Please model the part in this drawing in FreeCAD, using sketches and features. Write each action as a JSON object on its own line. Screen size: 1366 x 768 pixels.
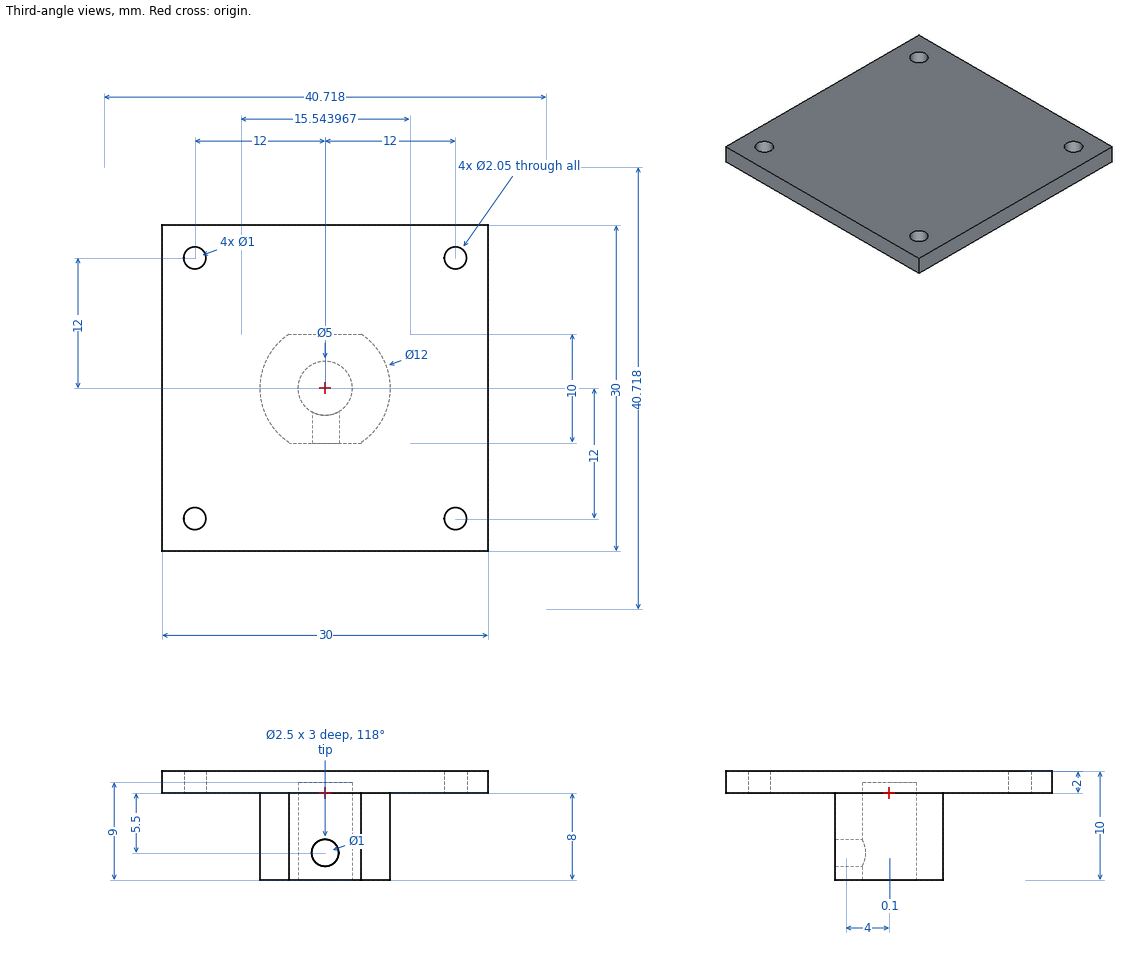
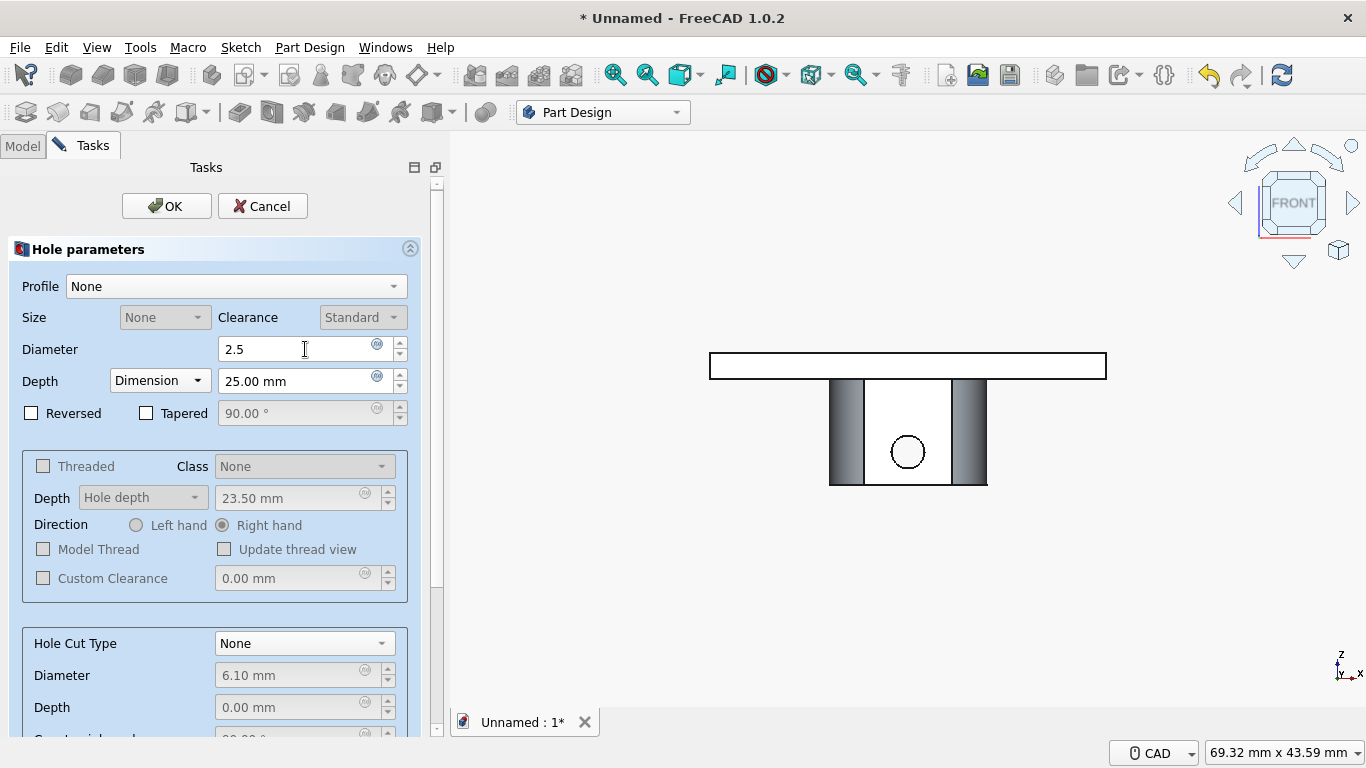
{"action": "triple_click", "coordinate": [305, 381]}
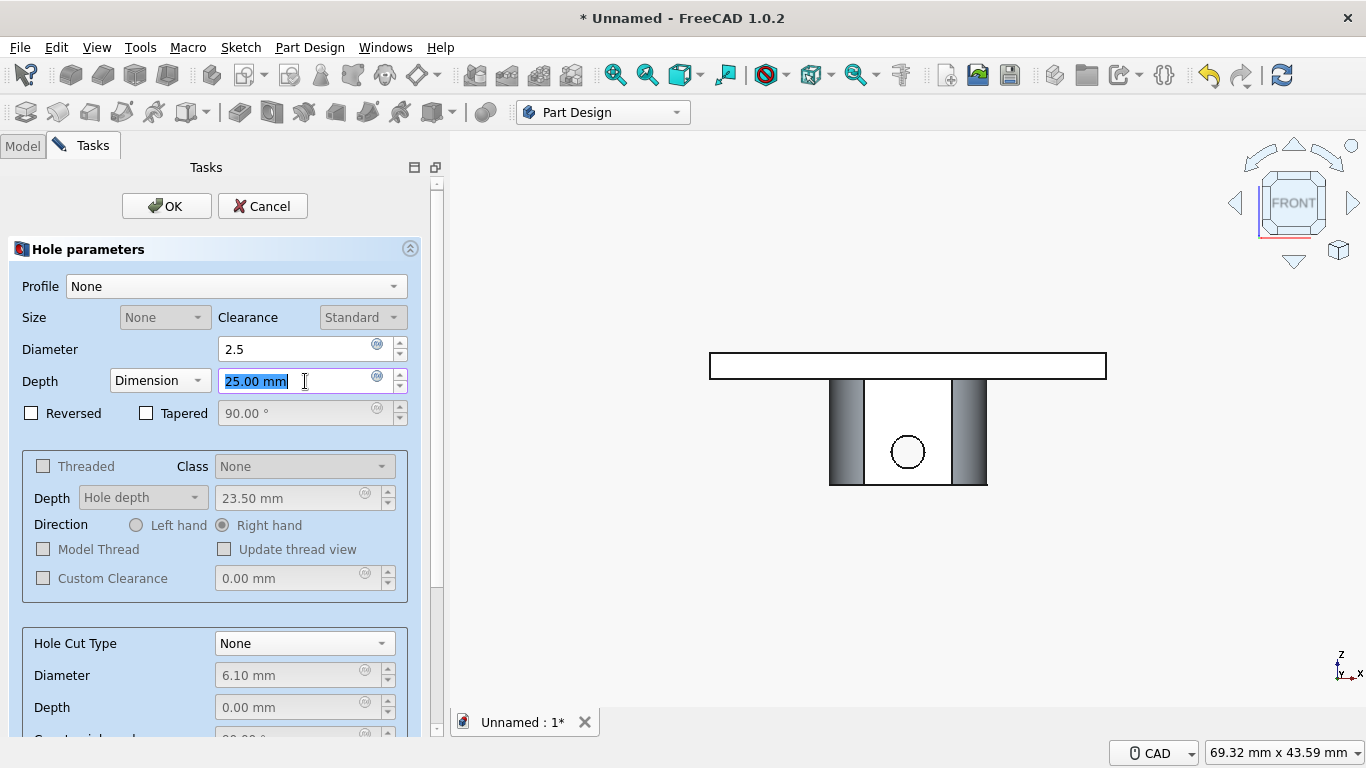
{"action": "type", "text": "3"}
{"action": "key", "text": "Tab"}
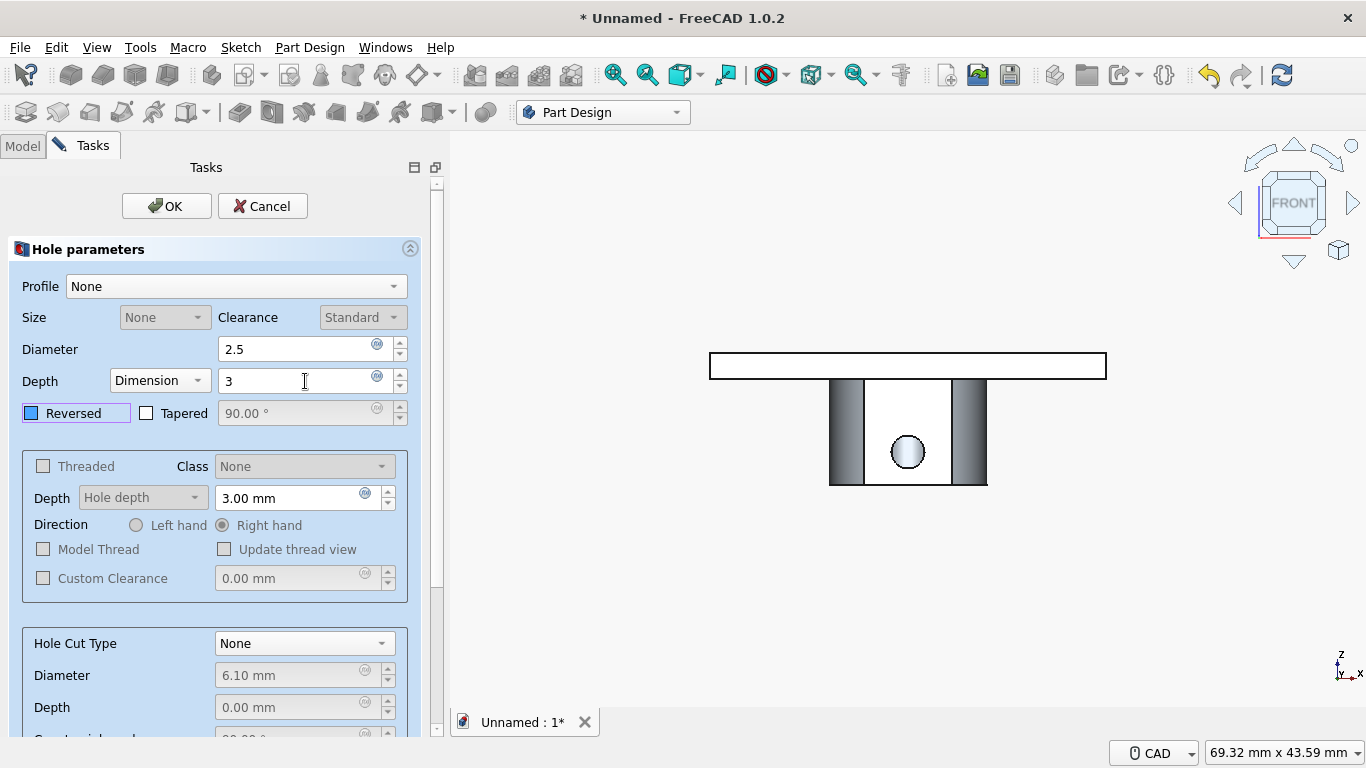
{"action": "left_click", "coordinate": [167, 206]}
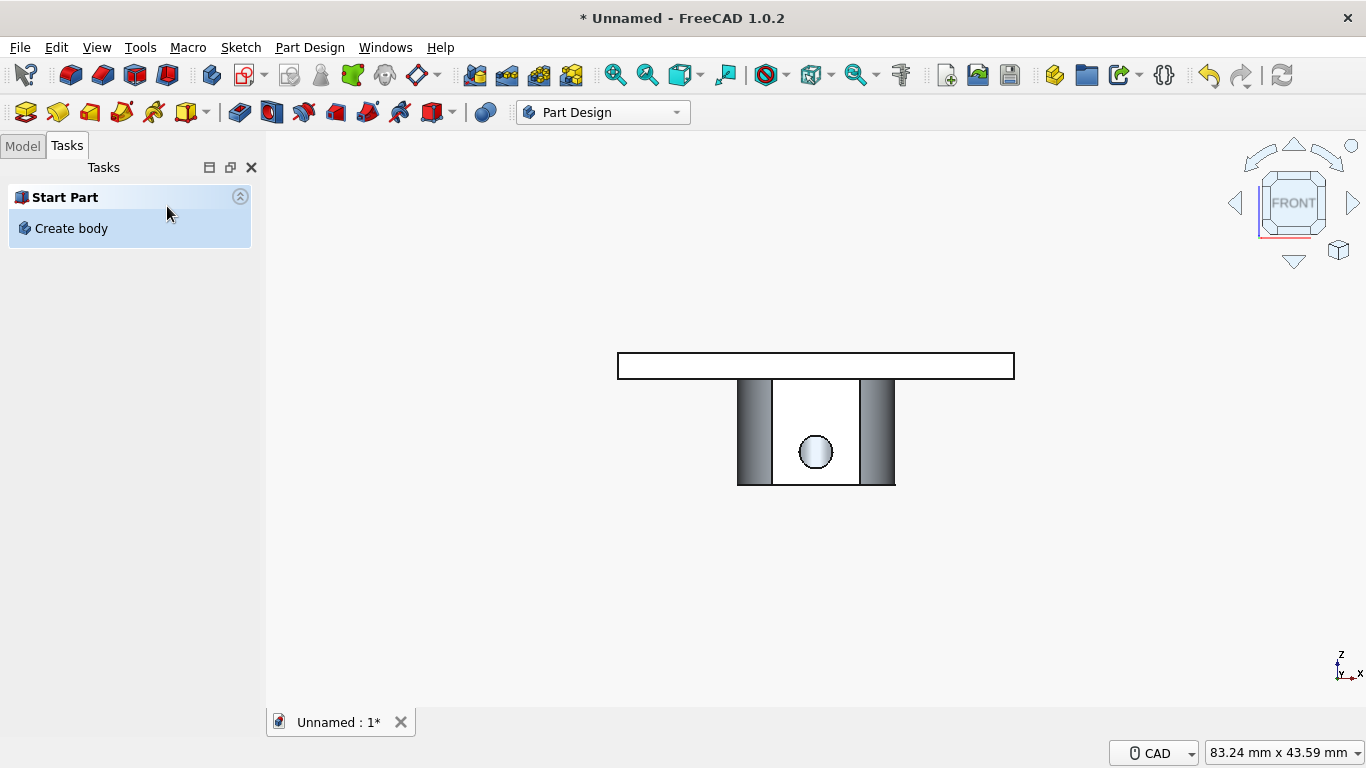
{"action": "key", "text": "v f"}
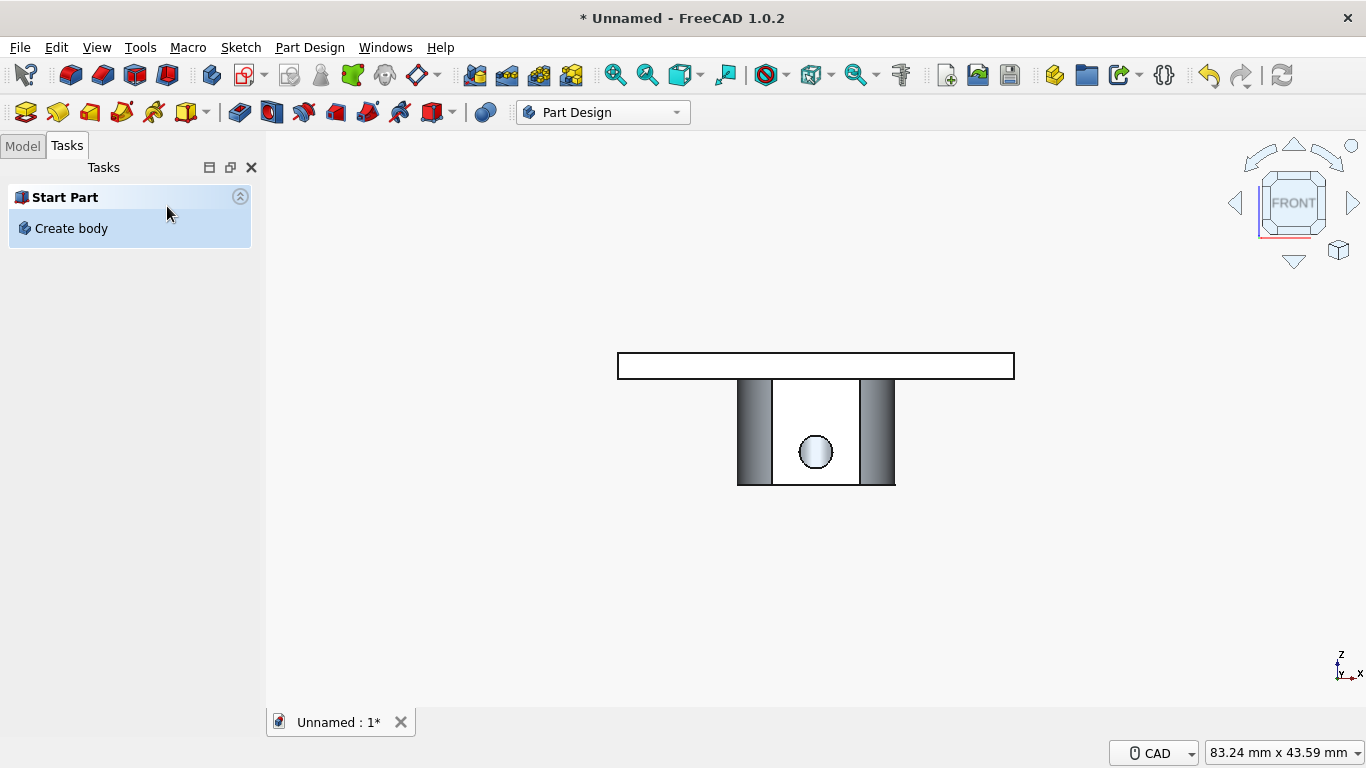
{"action": "key", "text": "0"}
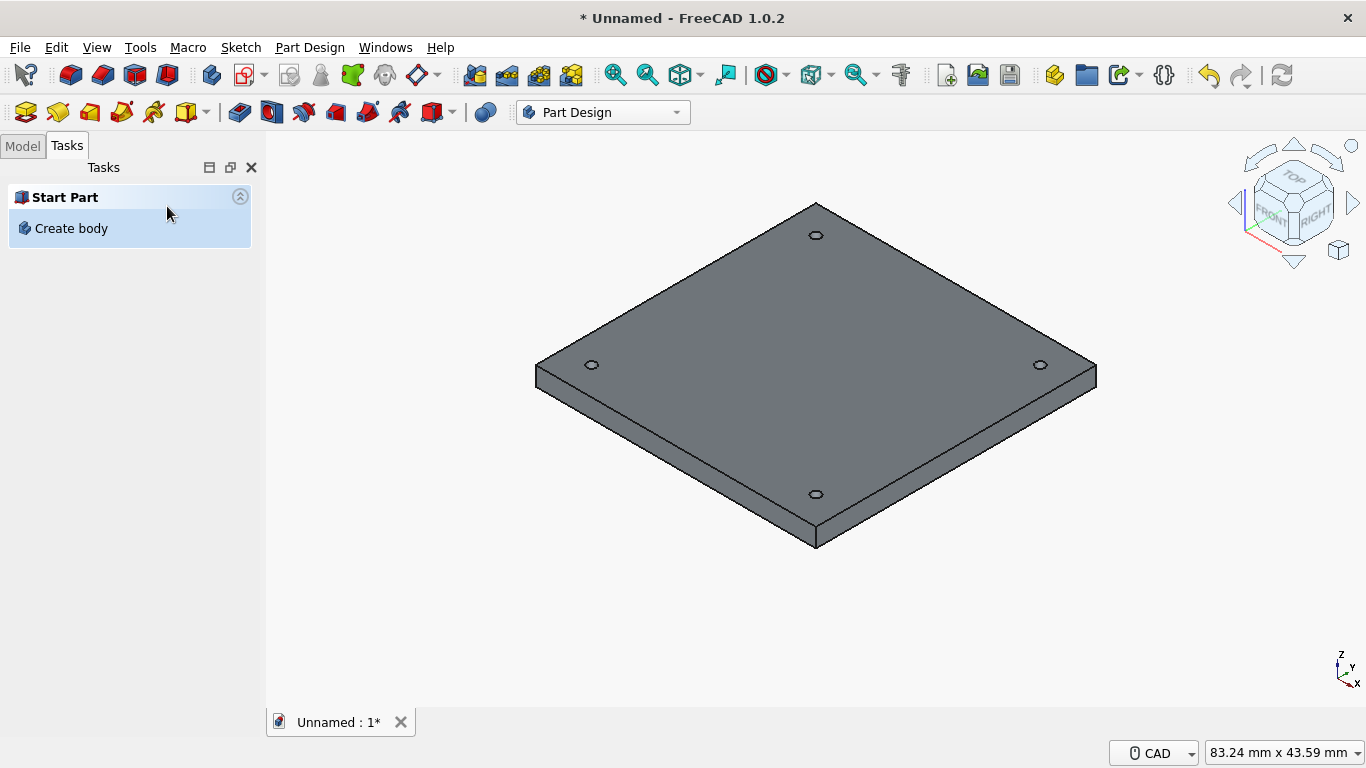
{"action": "left_click", "coordinate": [816, 364]}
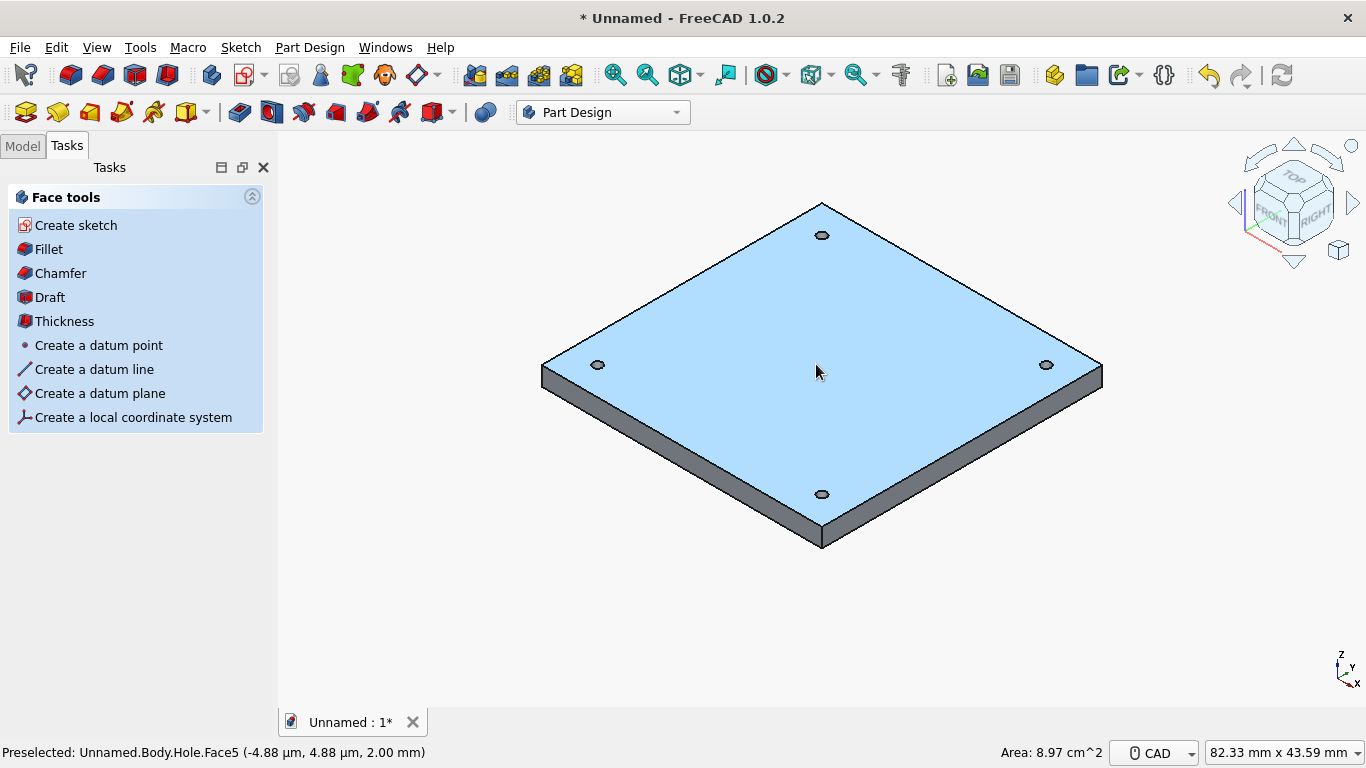
{"action": "left_click", "coordinate": [244, 76]}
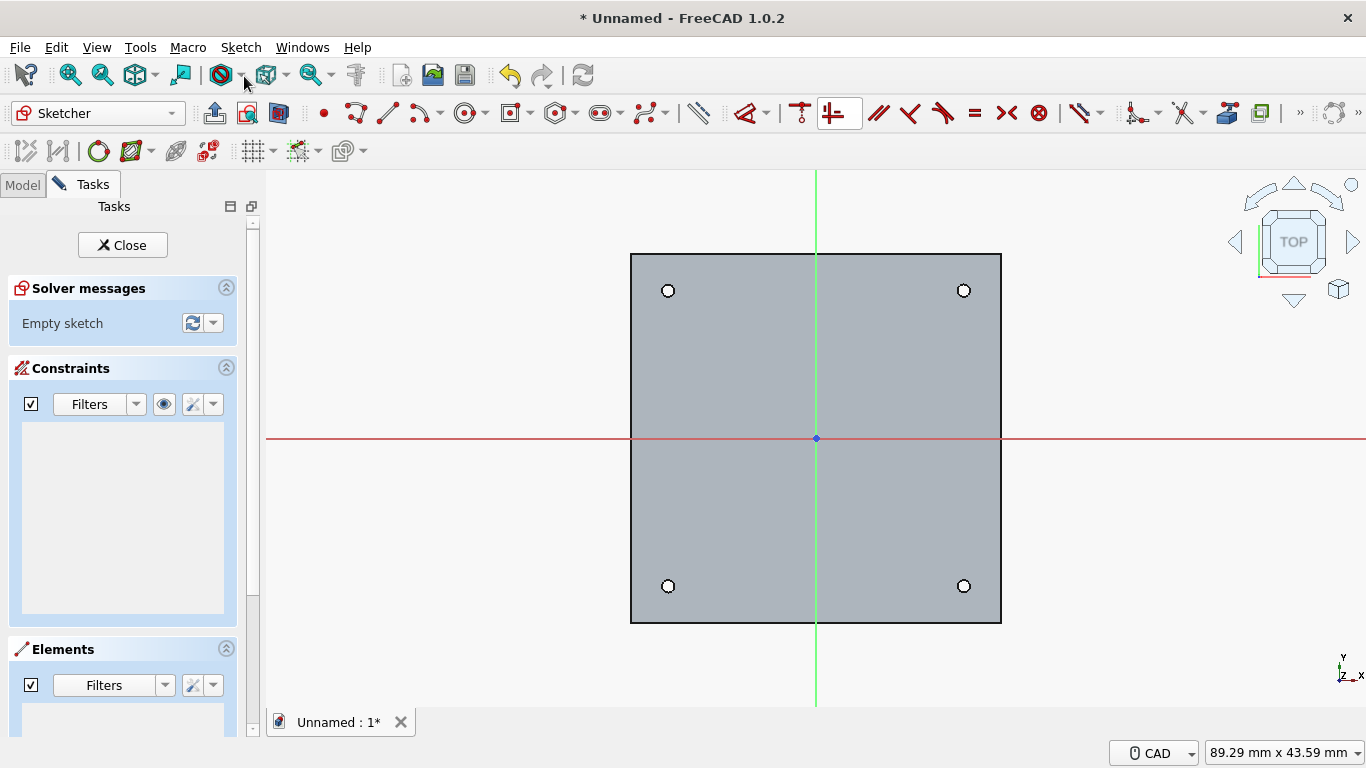
{"action": "left_click", "coordinate": [466, 114]}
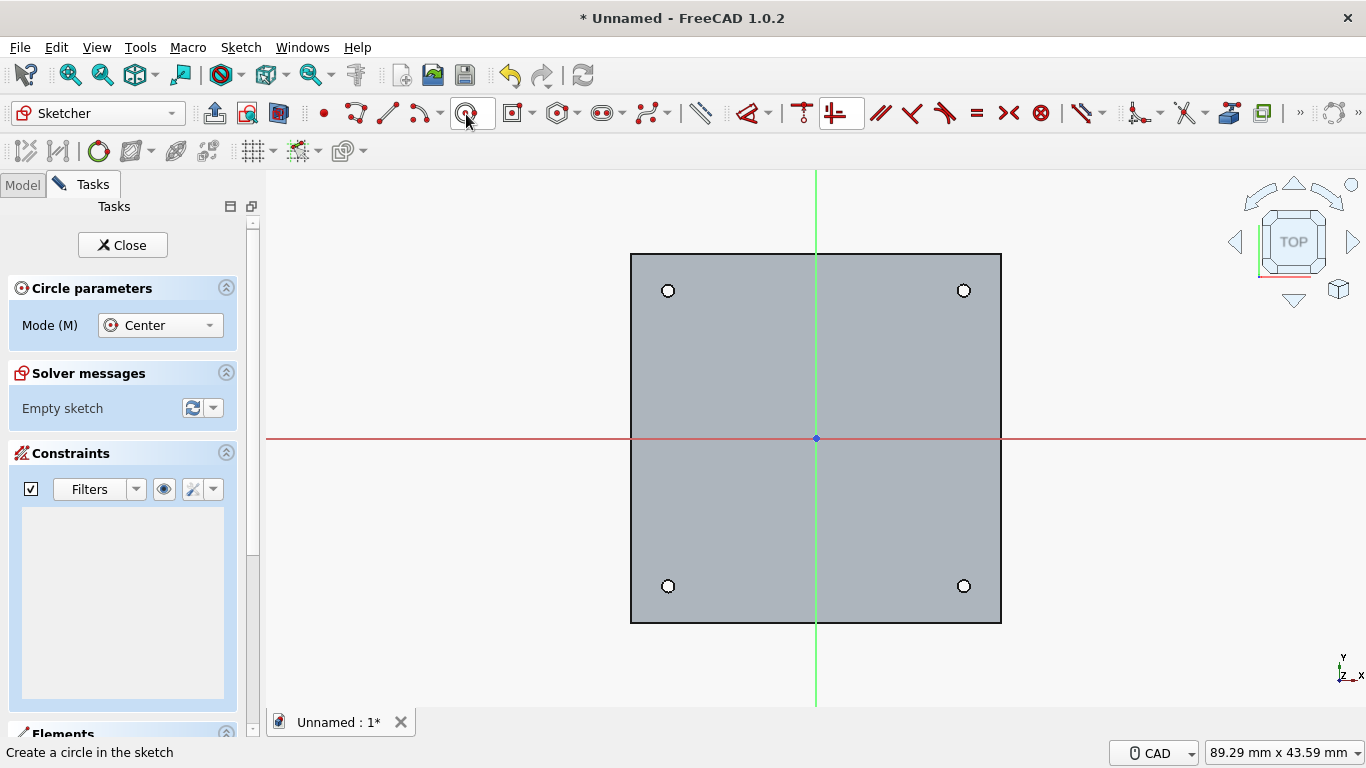
{"action": "scroll", "coordinate": [964, 291], "scroll_direction": "up", "scroll_amount": 3}